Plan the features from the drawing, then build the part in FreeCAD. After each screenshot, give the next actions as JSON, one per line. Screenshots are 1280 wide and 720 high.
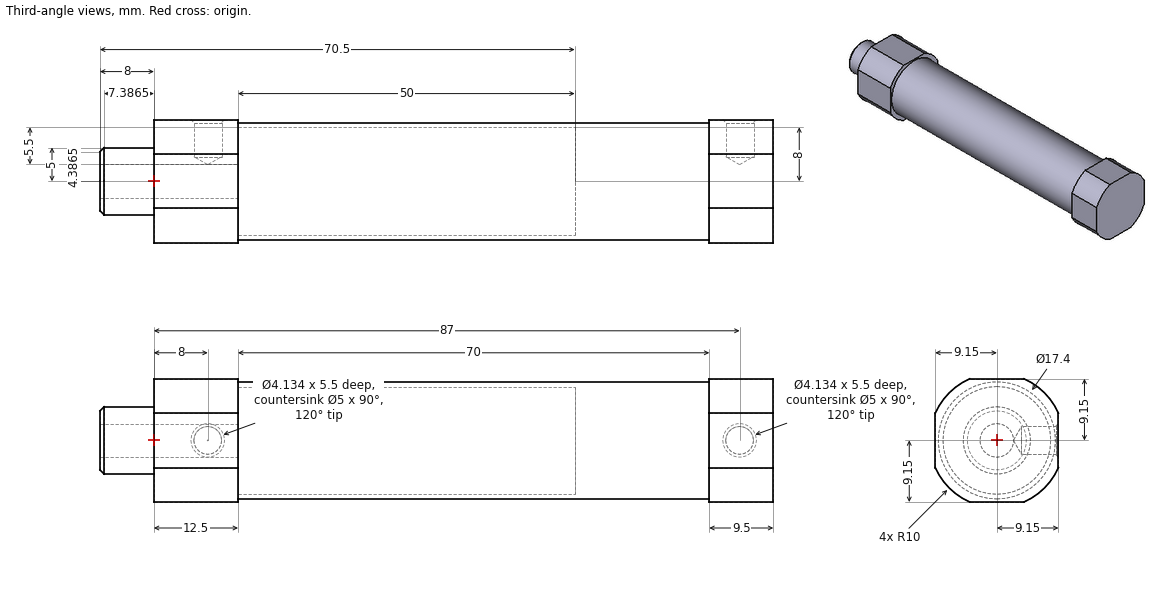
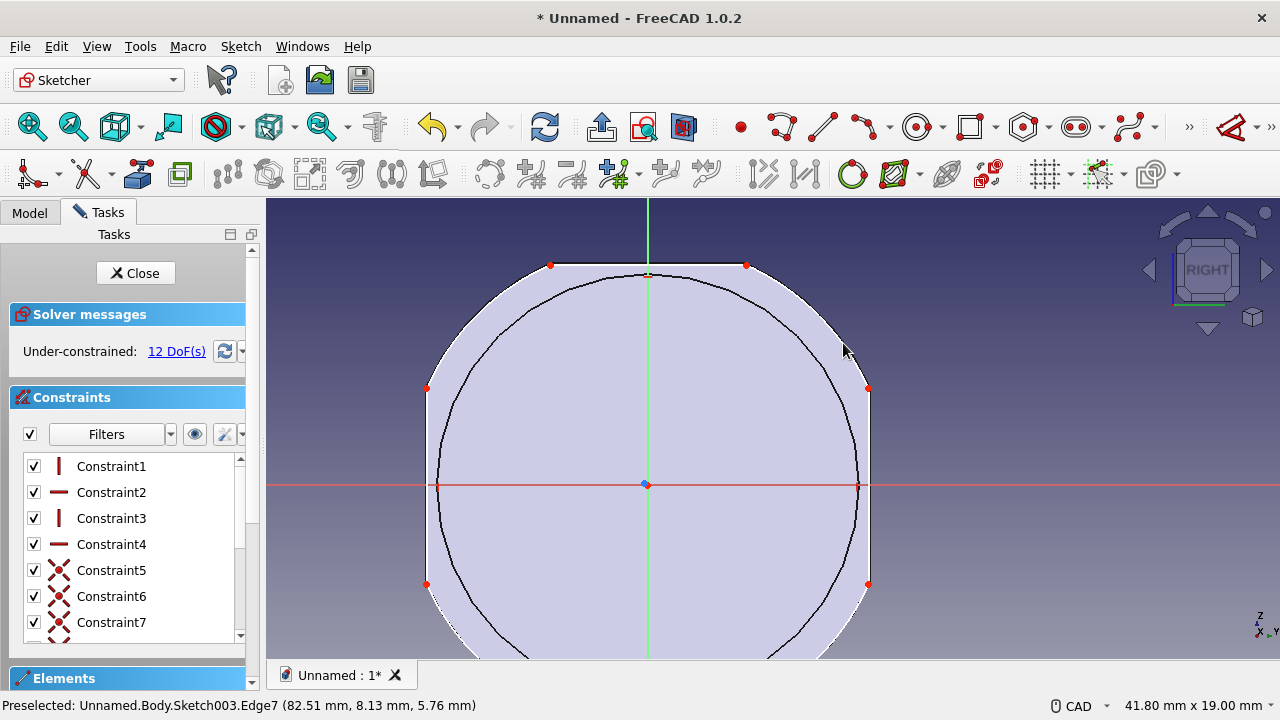
{"action": "left_click", "coordinate": [454, 630]}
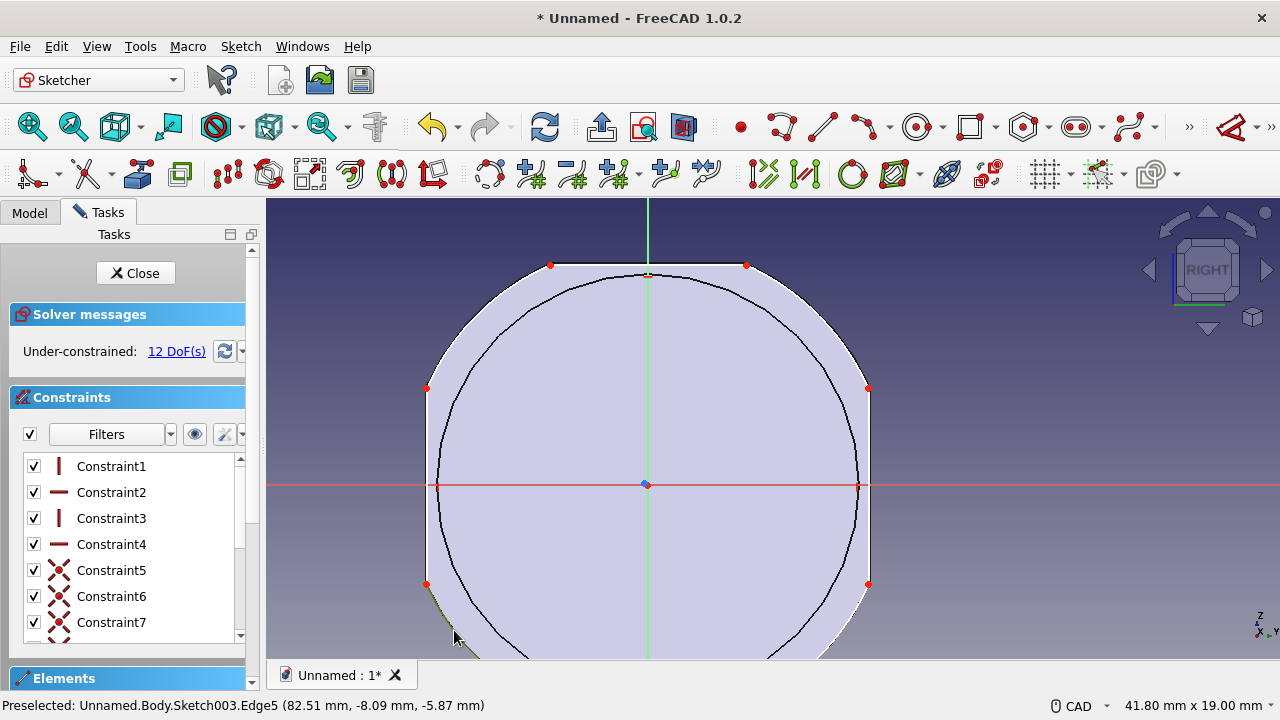
{"action": "left_click", "coordinate": [504, 292]}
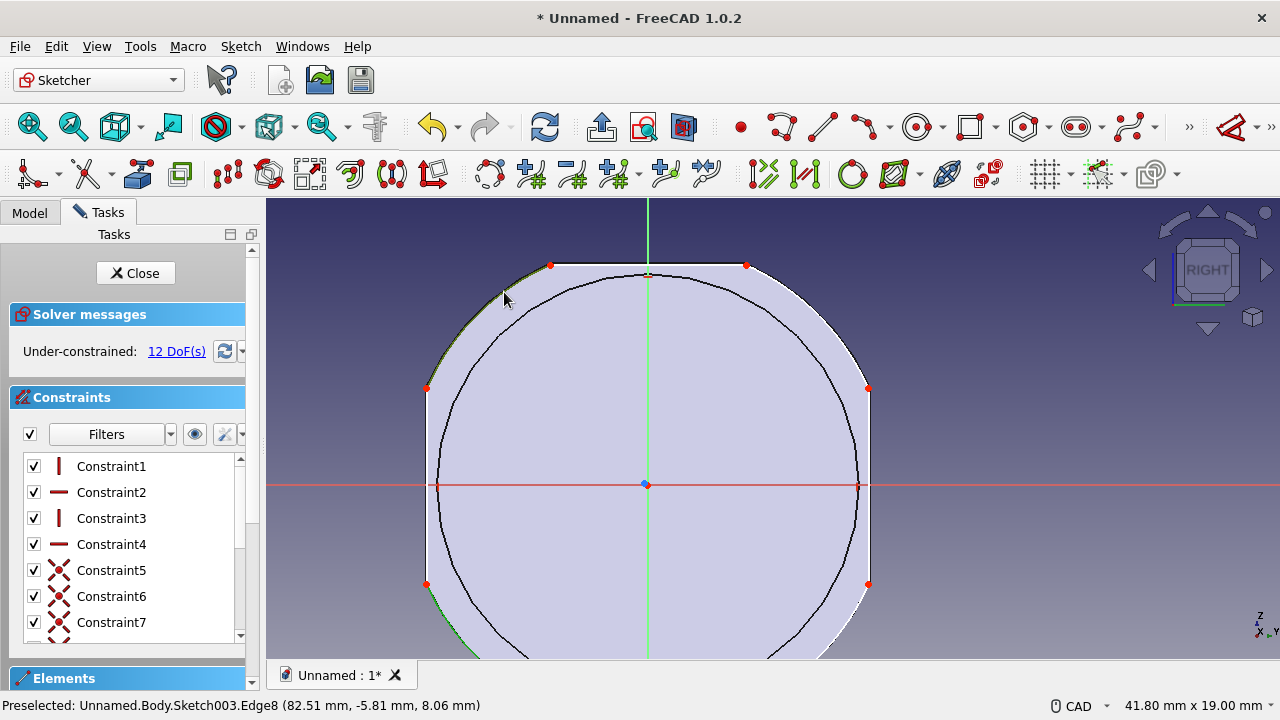
{"action": "key", "text": "c"}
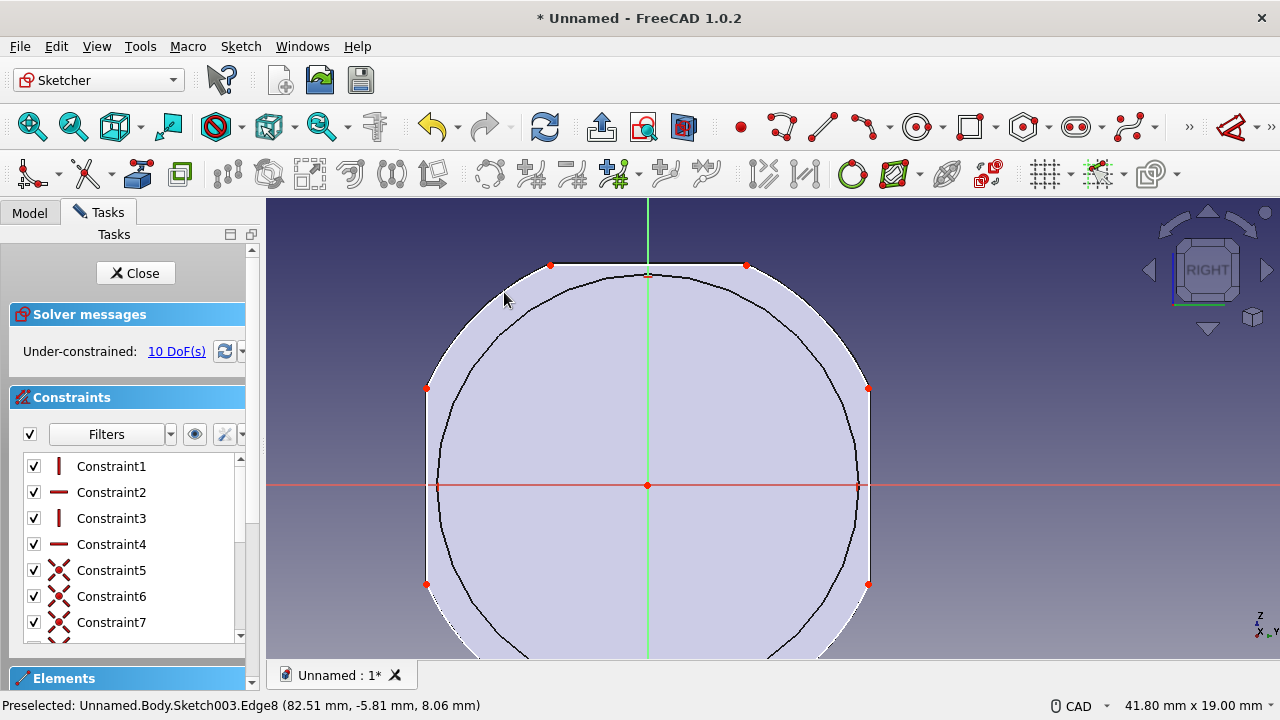
{"action": "left_click_drag", "start_coordinate": [637, 475], "coordinate": [658, 495]}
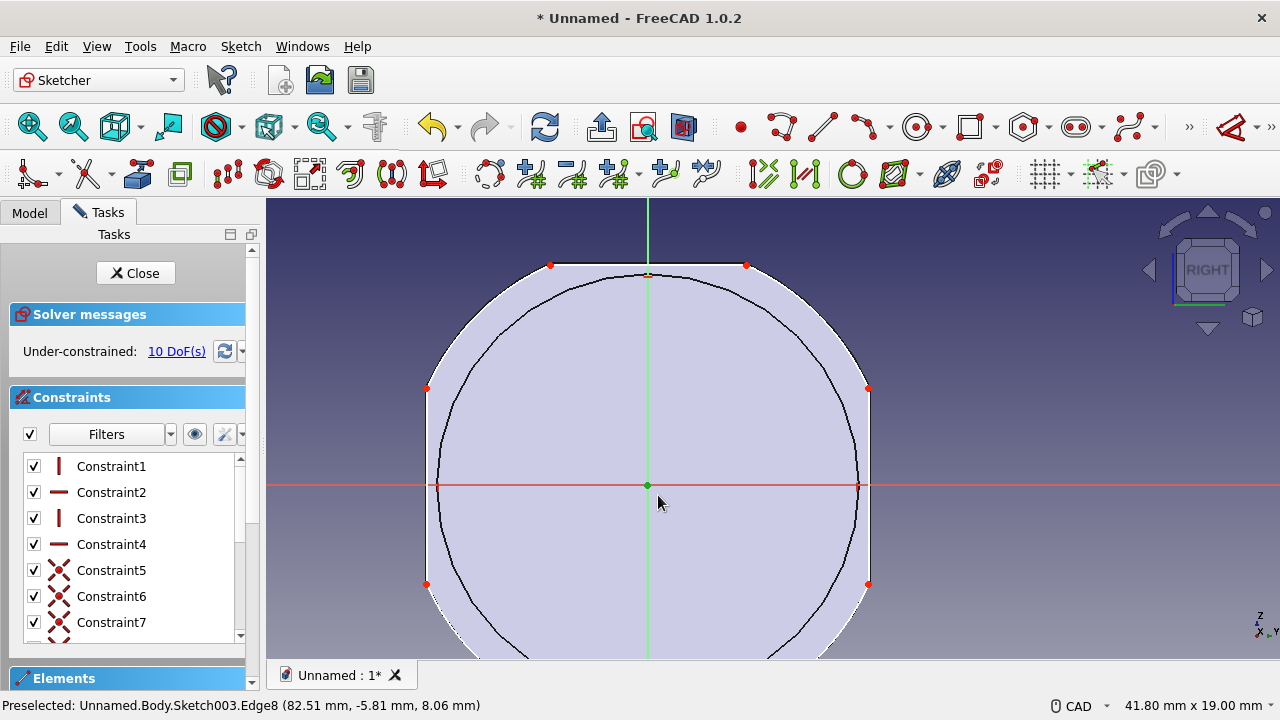
{"action": "key", "text": "c"}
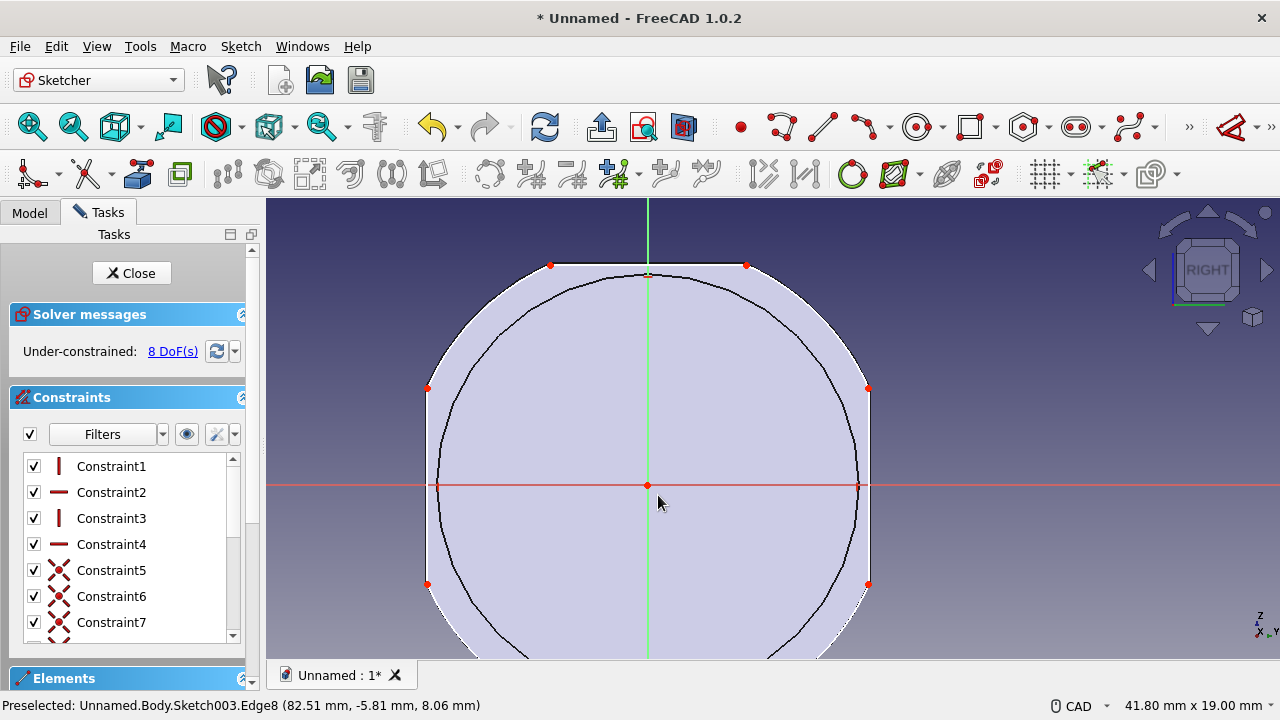
{"action": "left_click", "coordinate": [454, 630]}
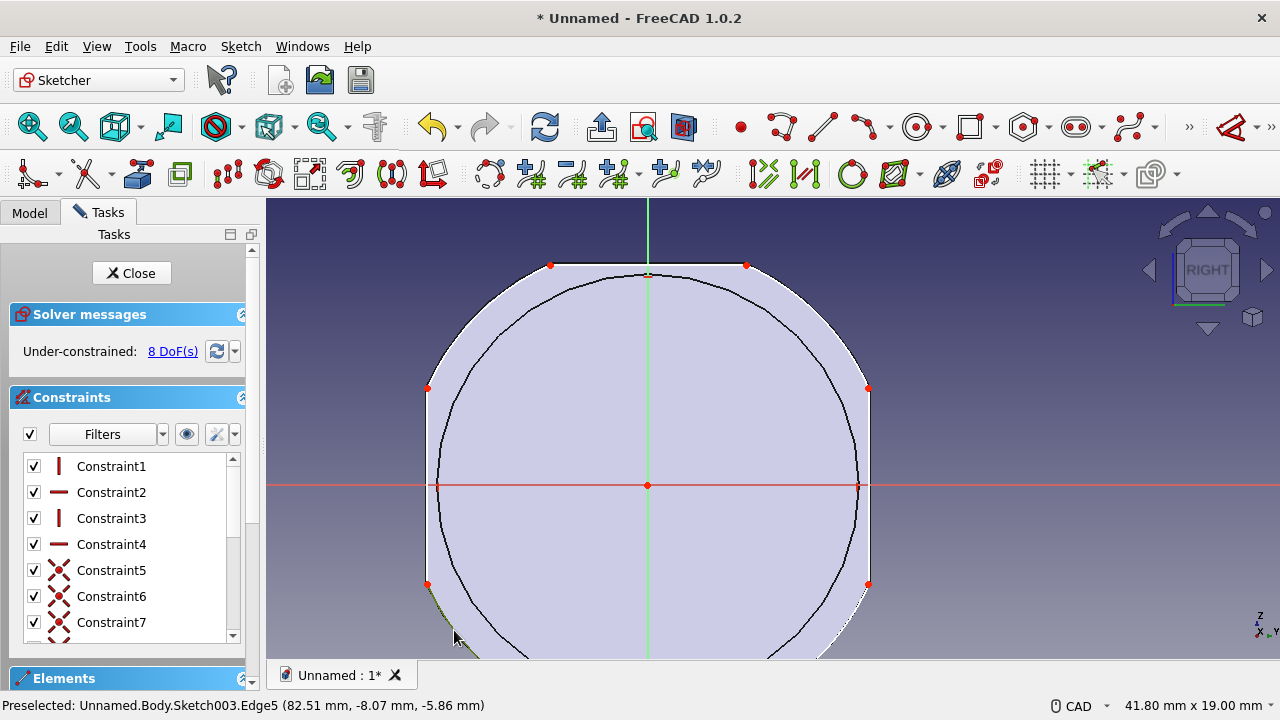
{"action": "left_click", "coordinate": [842, 630]}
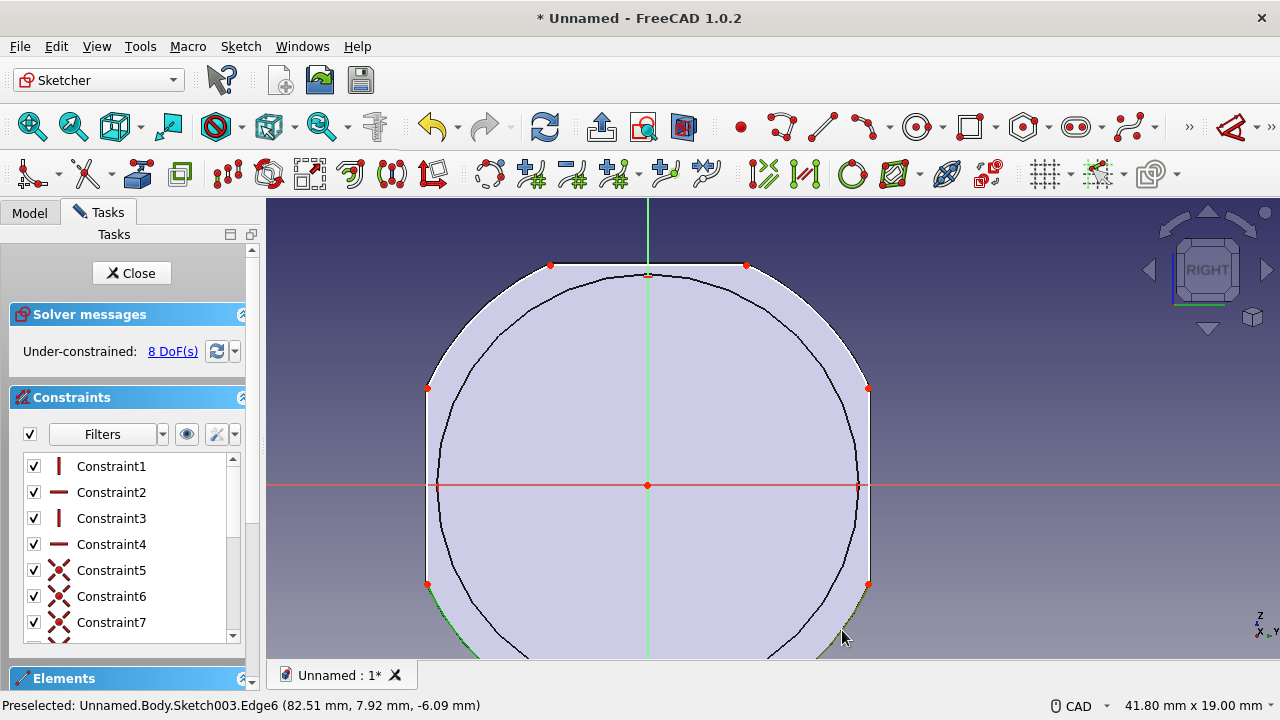
{"action": "left_click", "coordinate": [842, 343]}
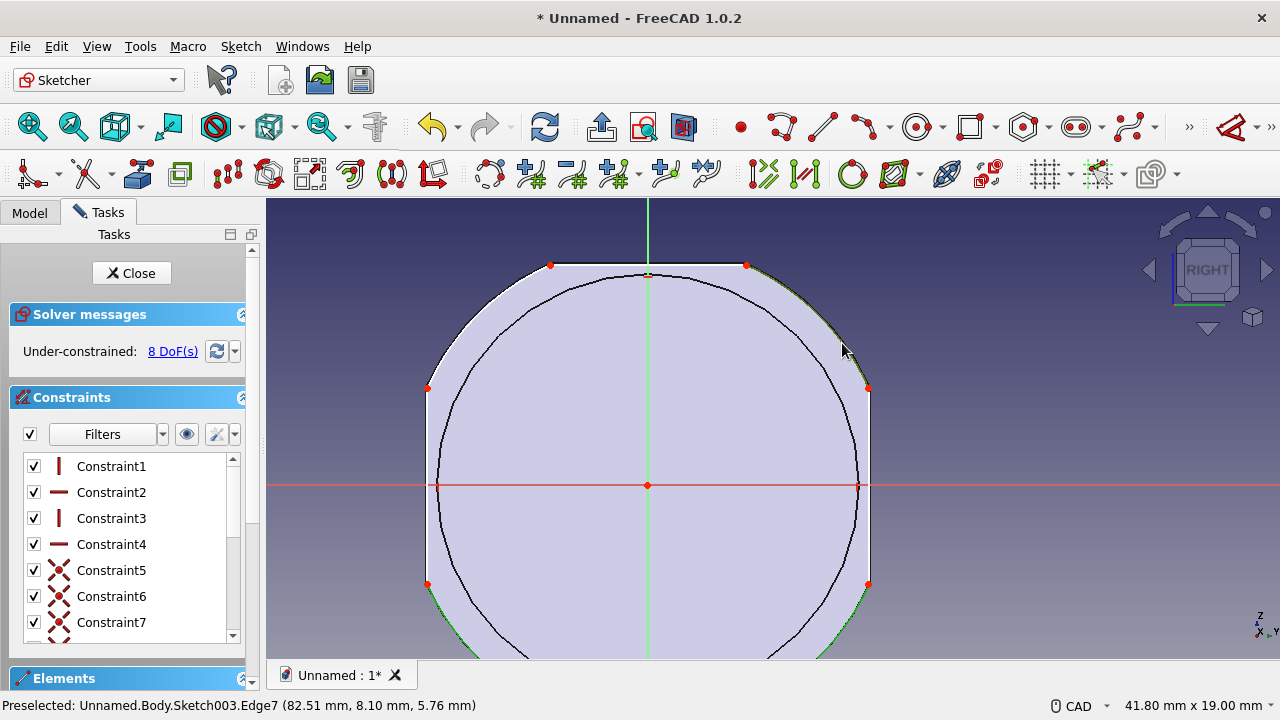
{"action": "left_click", "coordinate": [504, 292]}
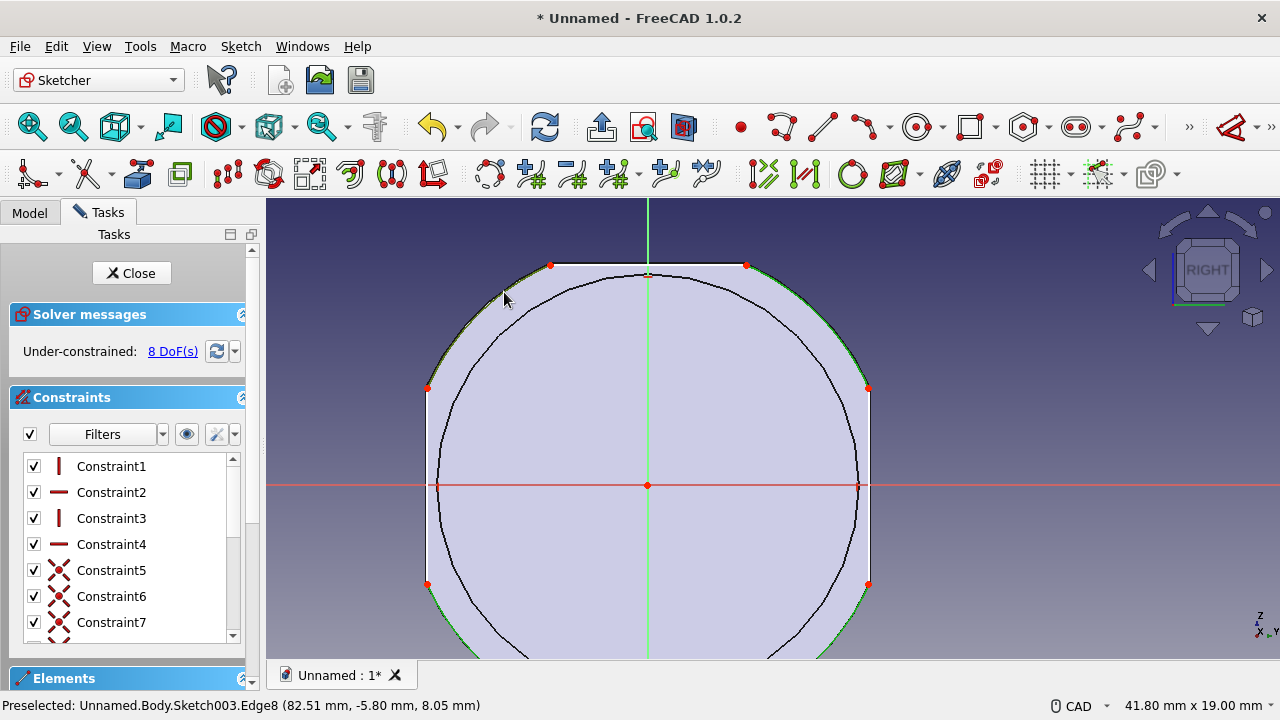
{"action": "key", "text": "e"}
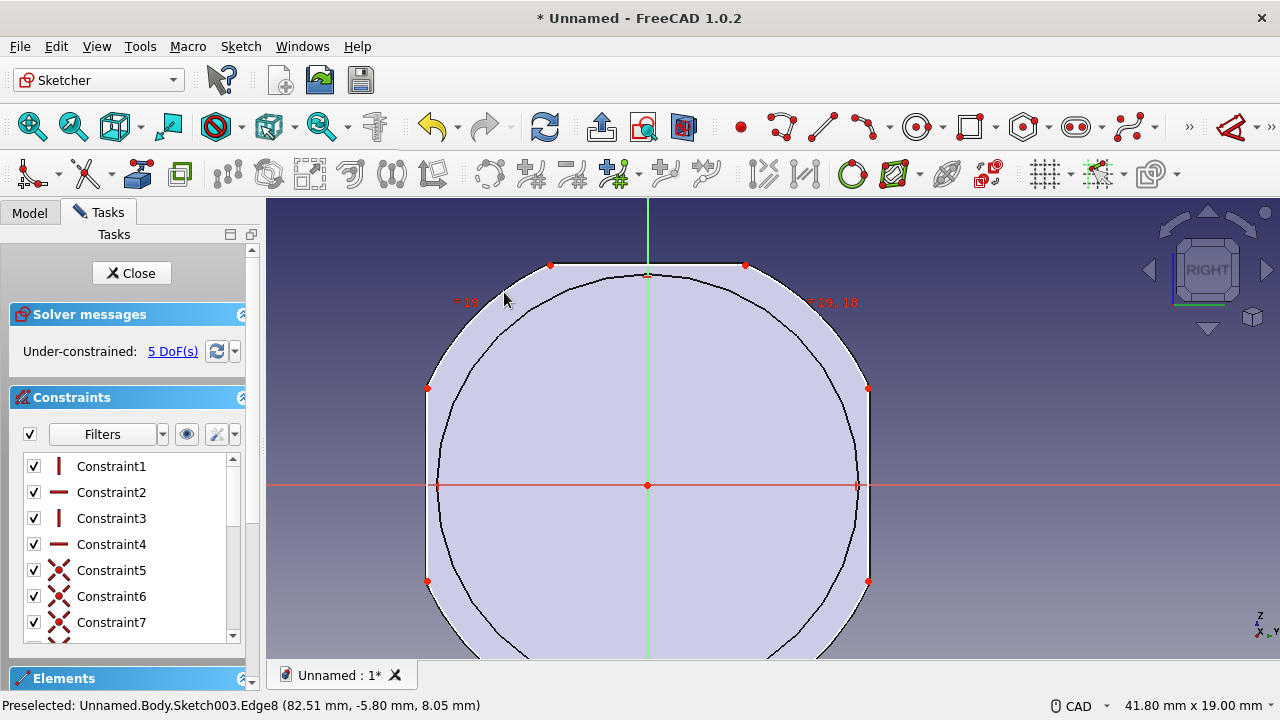
{"action": "left_click", "coordinate": [1230, 128]}